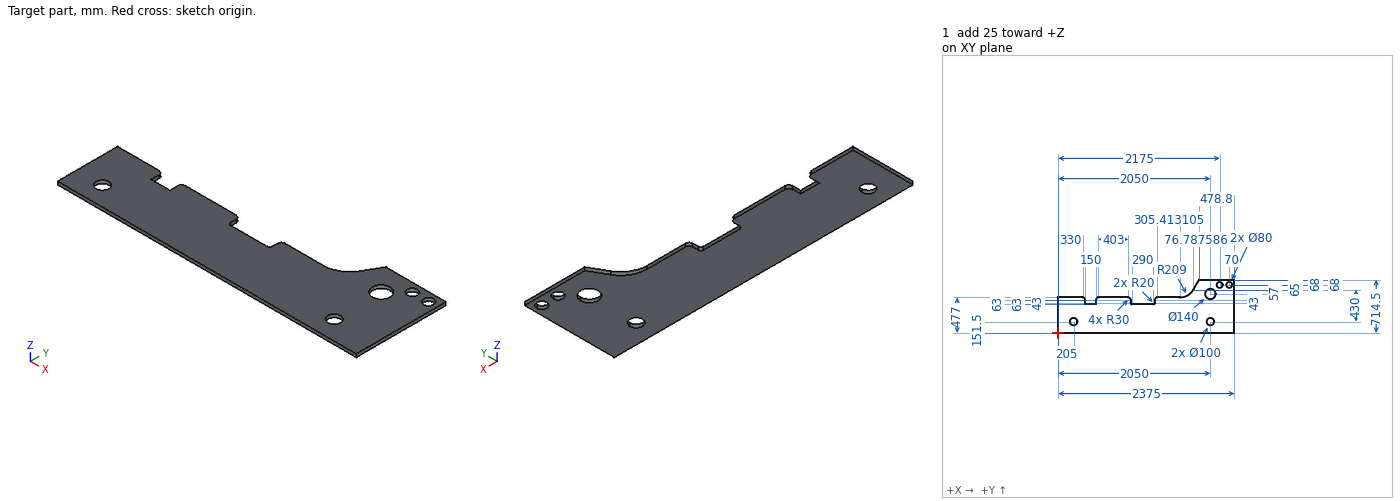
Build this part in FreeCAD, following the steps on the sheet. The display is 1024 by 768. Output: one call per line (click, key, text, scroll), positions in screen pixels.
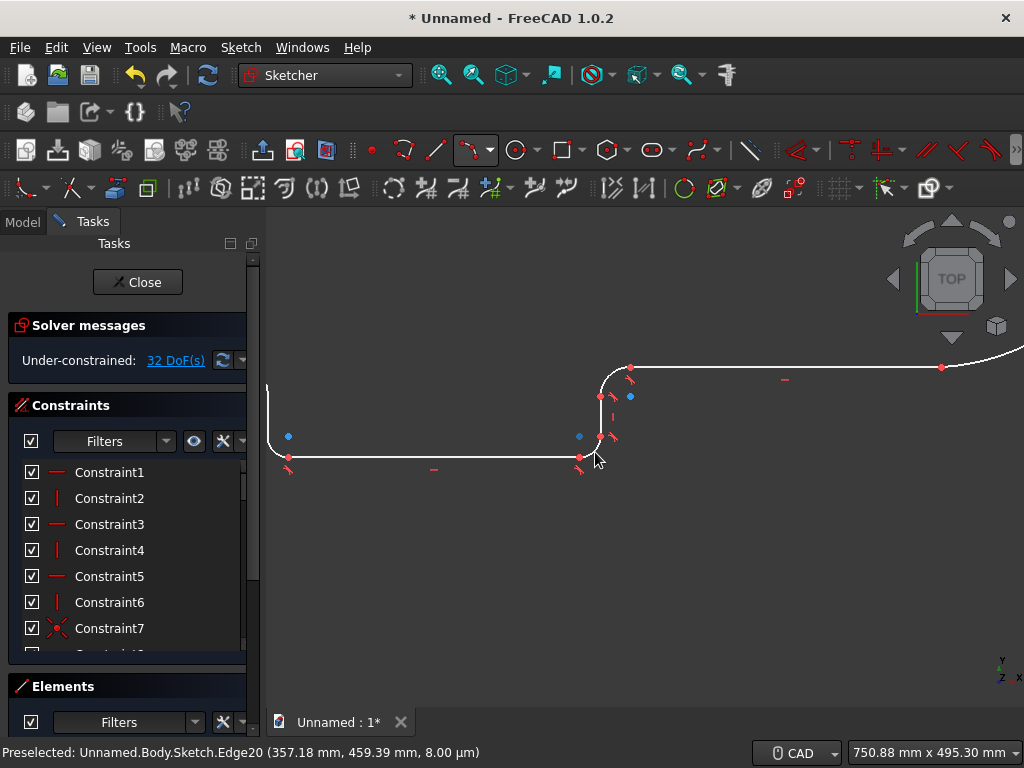
click(594, 451)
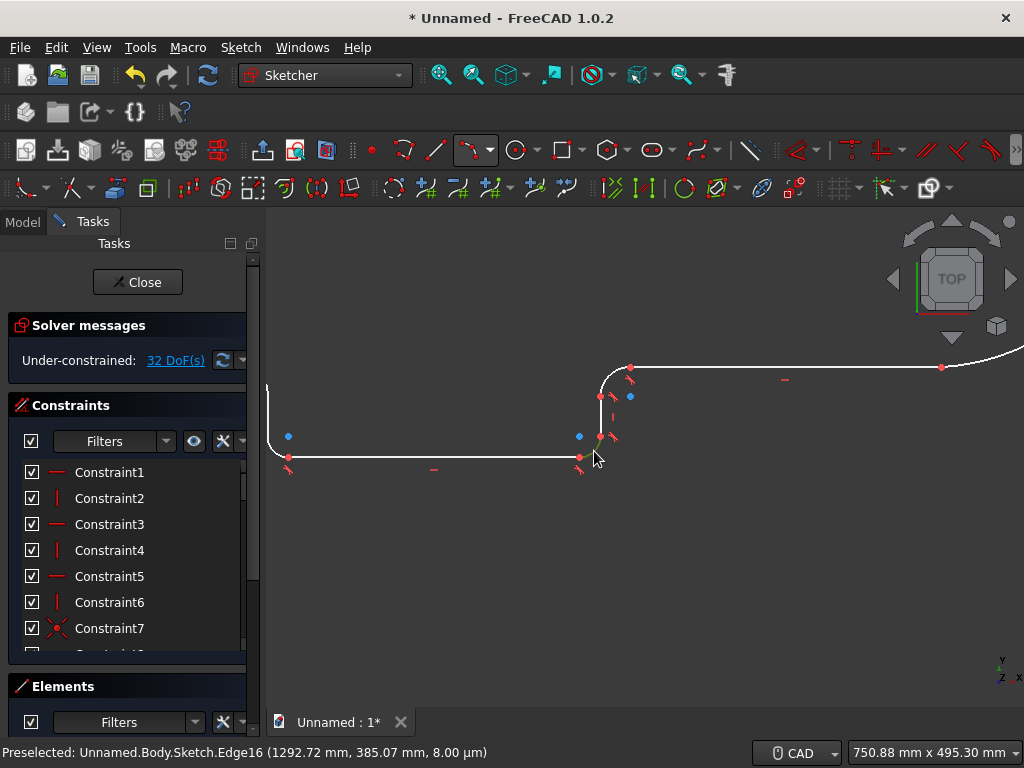
scroll(595, 452, down, 9)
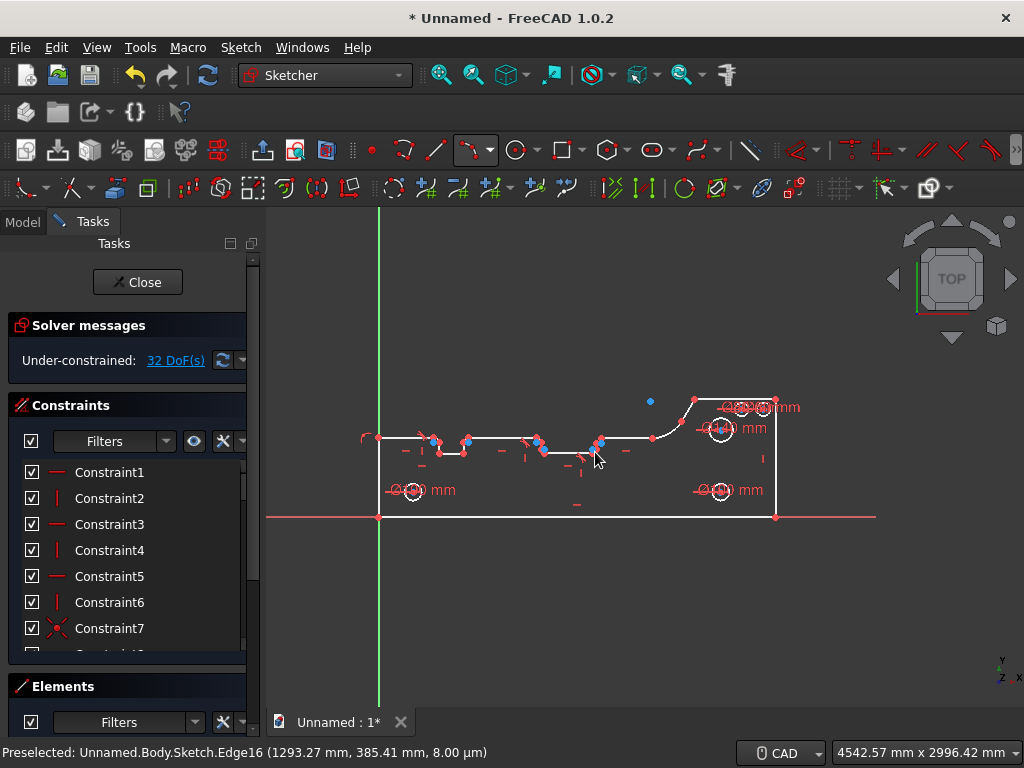
scroll(542, 451, up, 11)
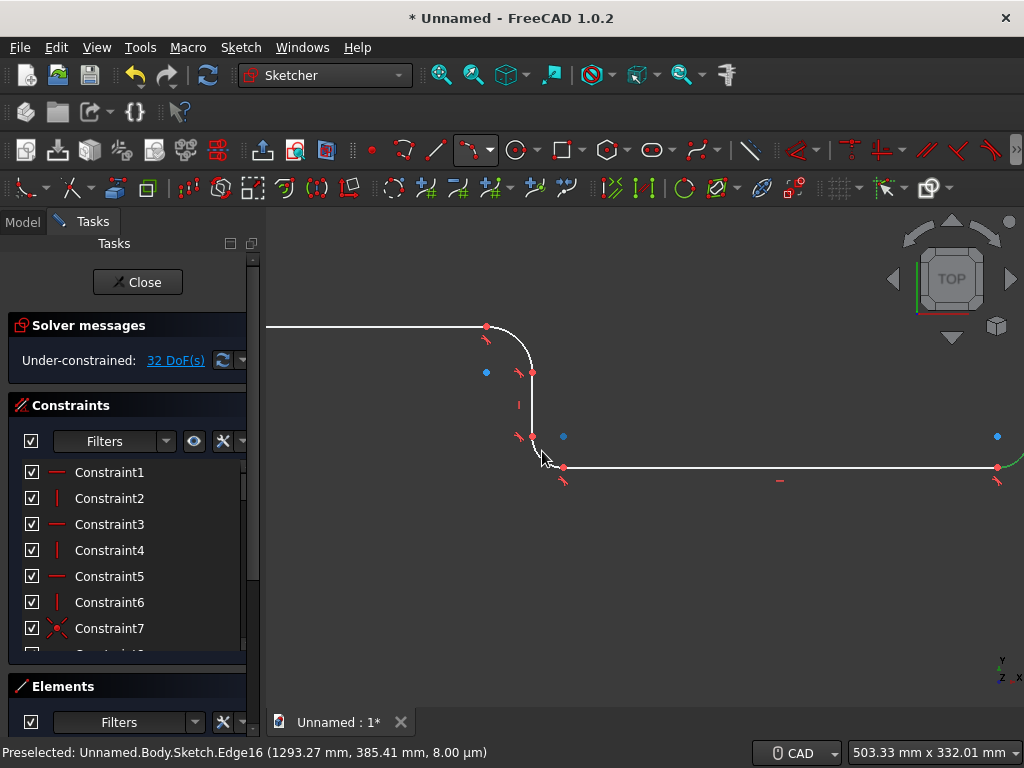
click(536, 451)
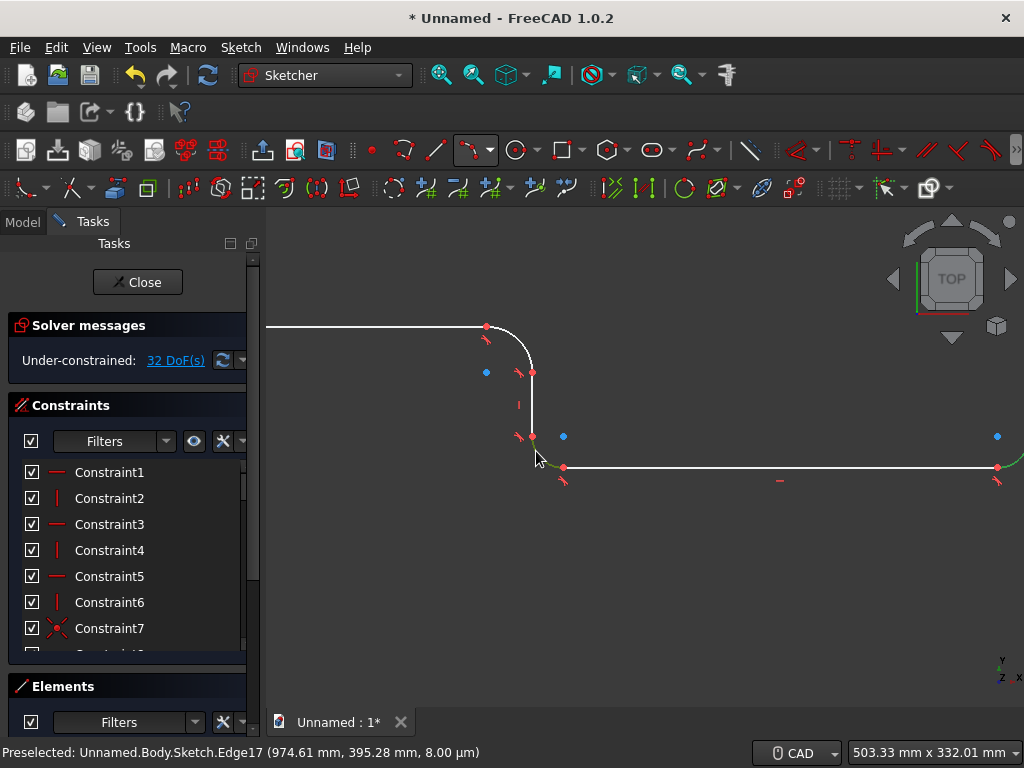
key(e)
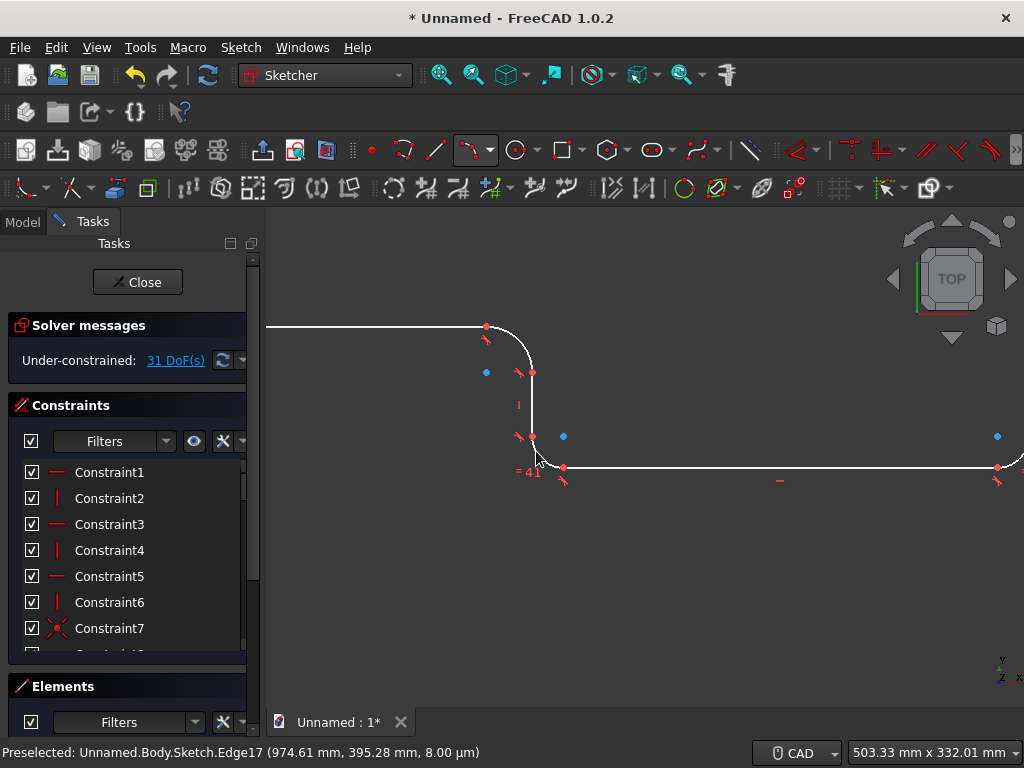
scroll(542, 451, down, 11)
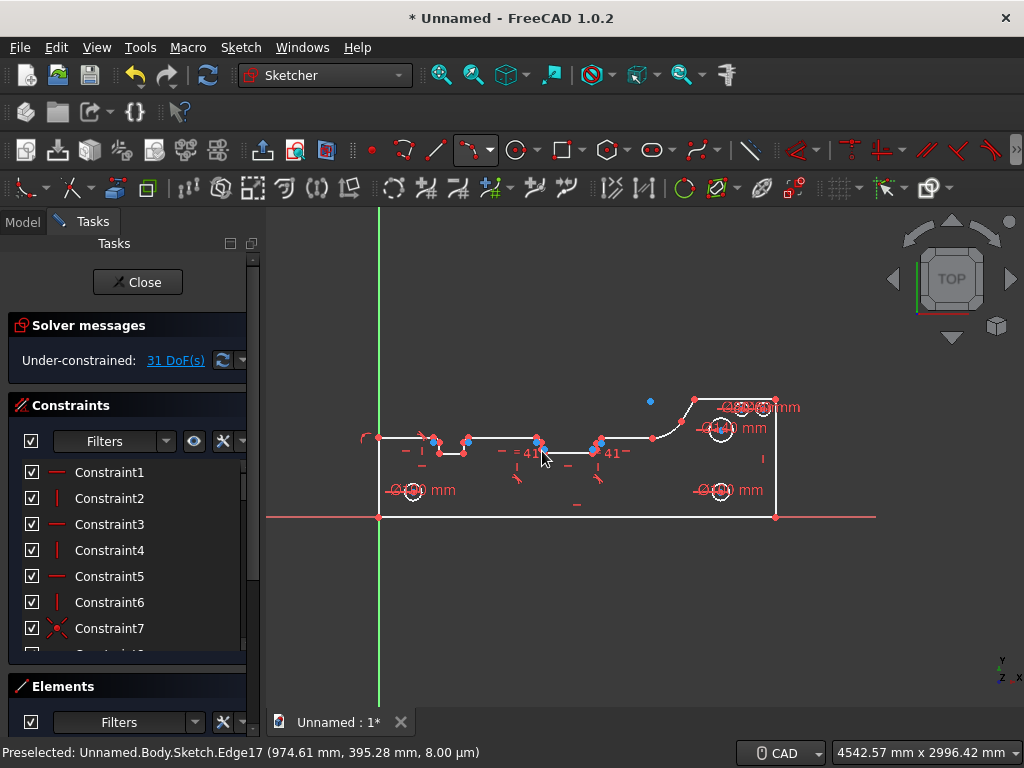
scroll(599, 439, up, 9)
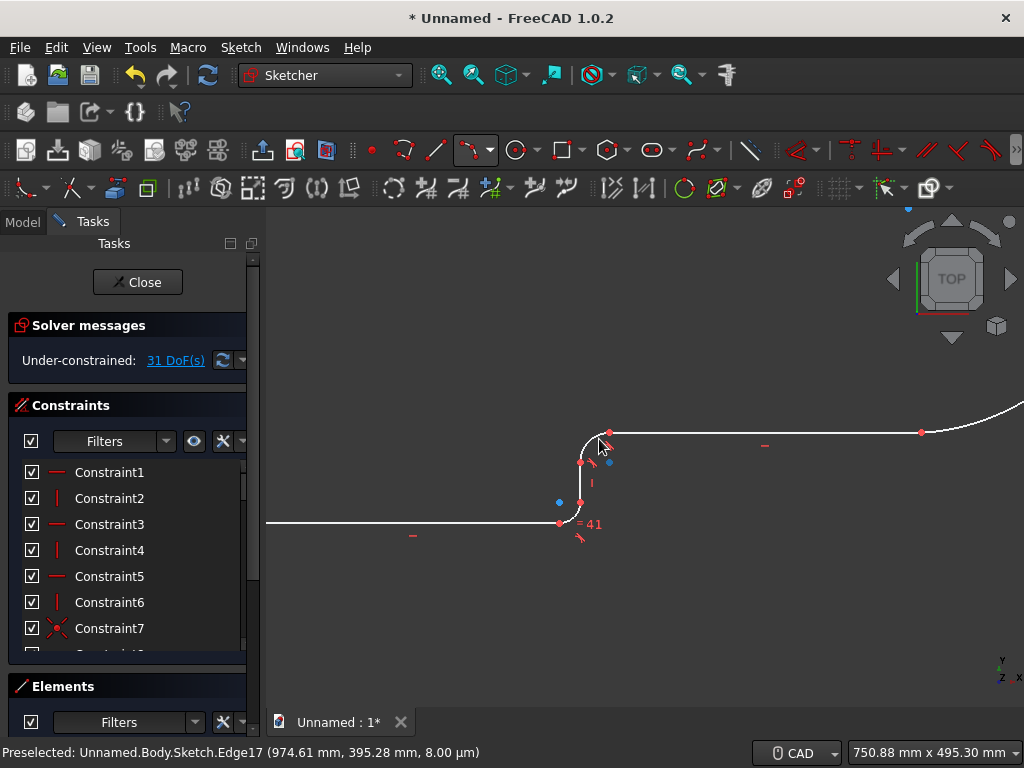
click(597, 436)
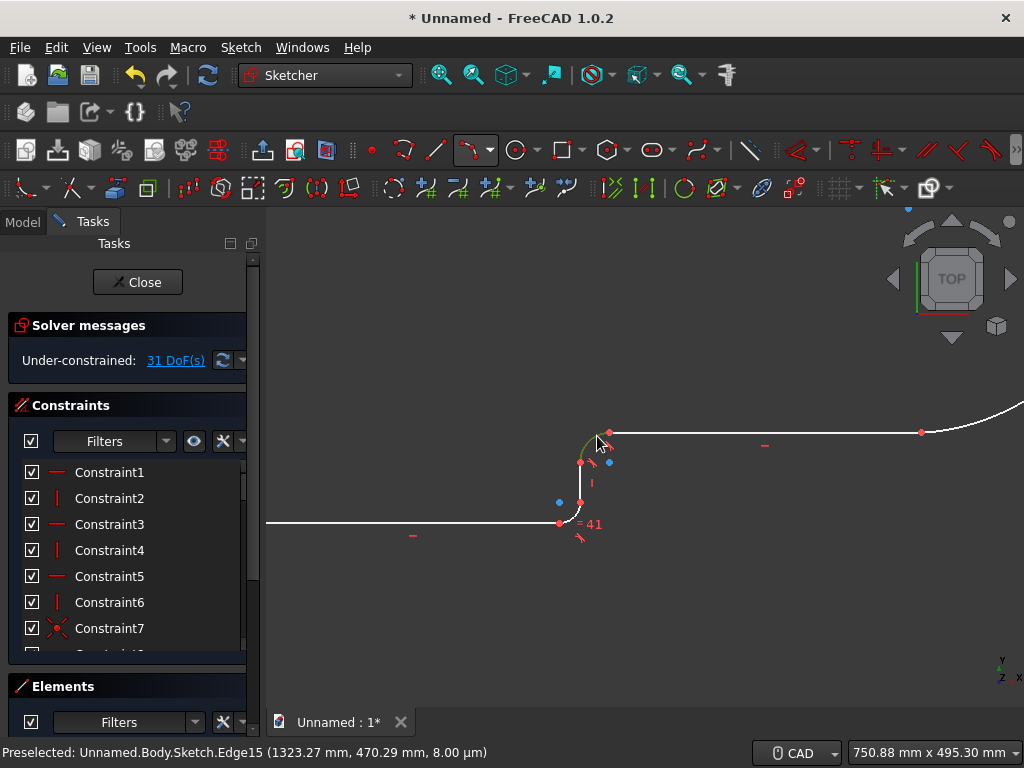
scroll(599, 439, down, 9)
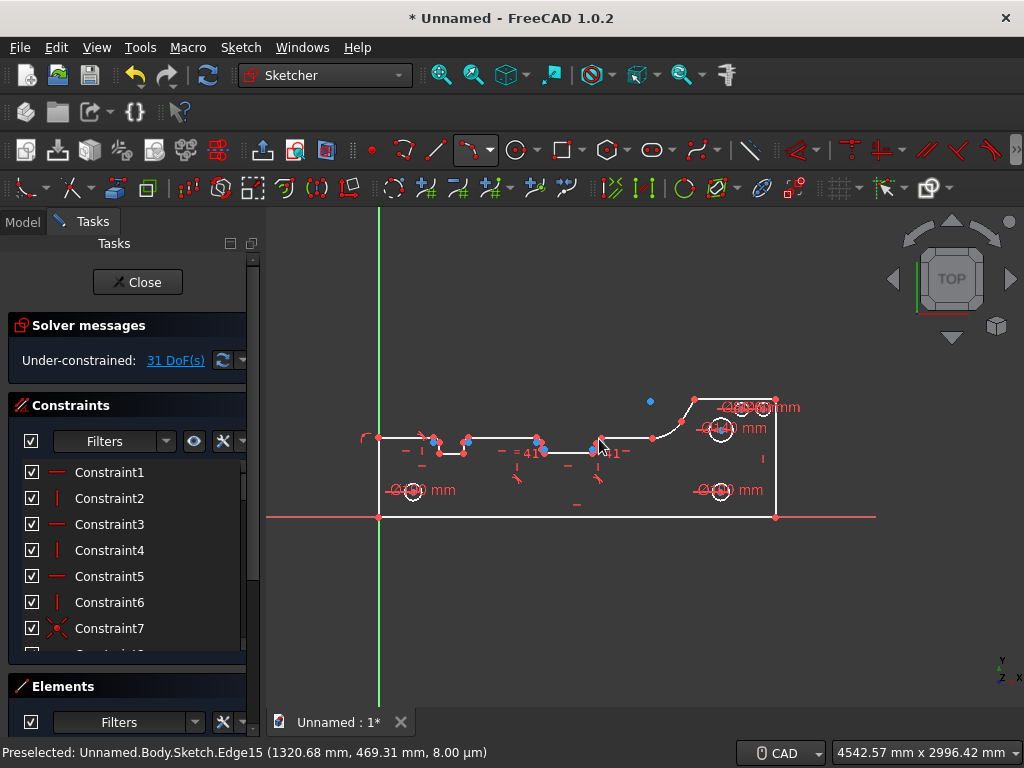
scroll(541, 440, up, 9)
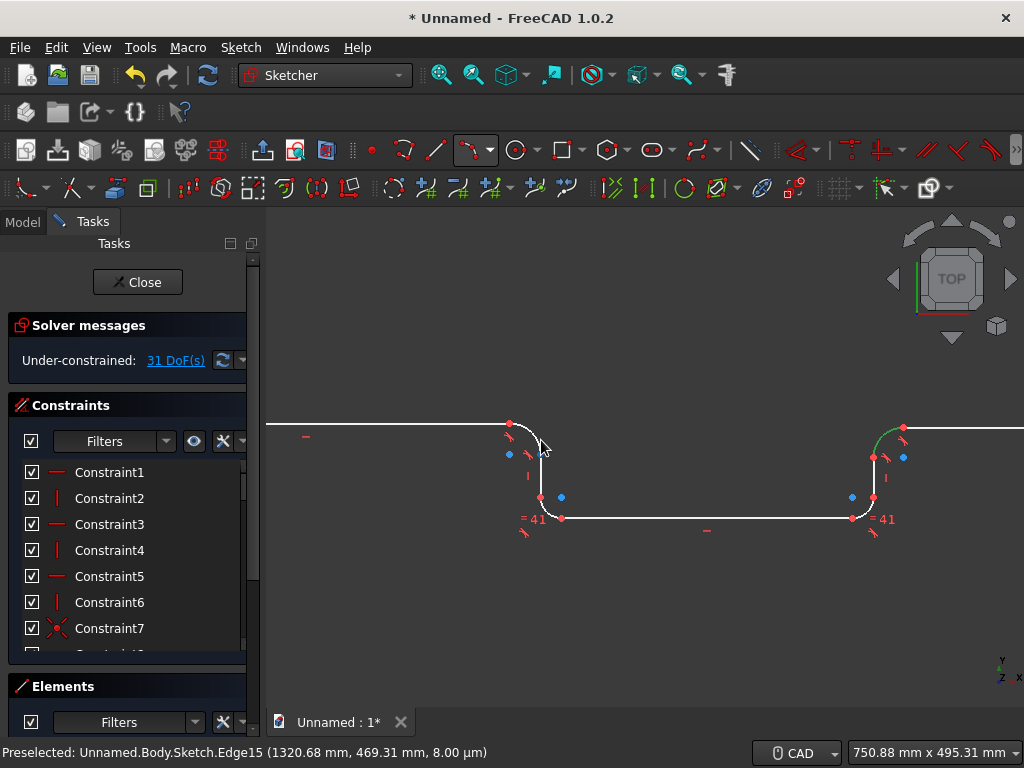
click(537, 440)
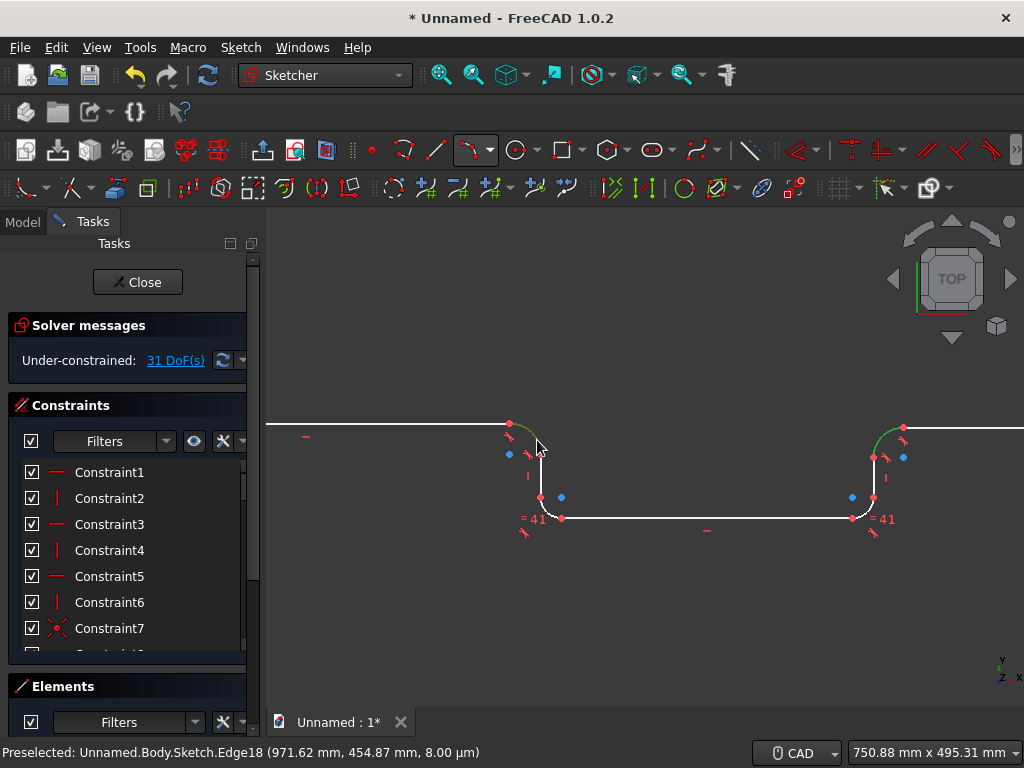
scroll(541, 440, down, 9)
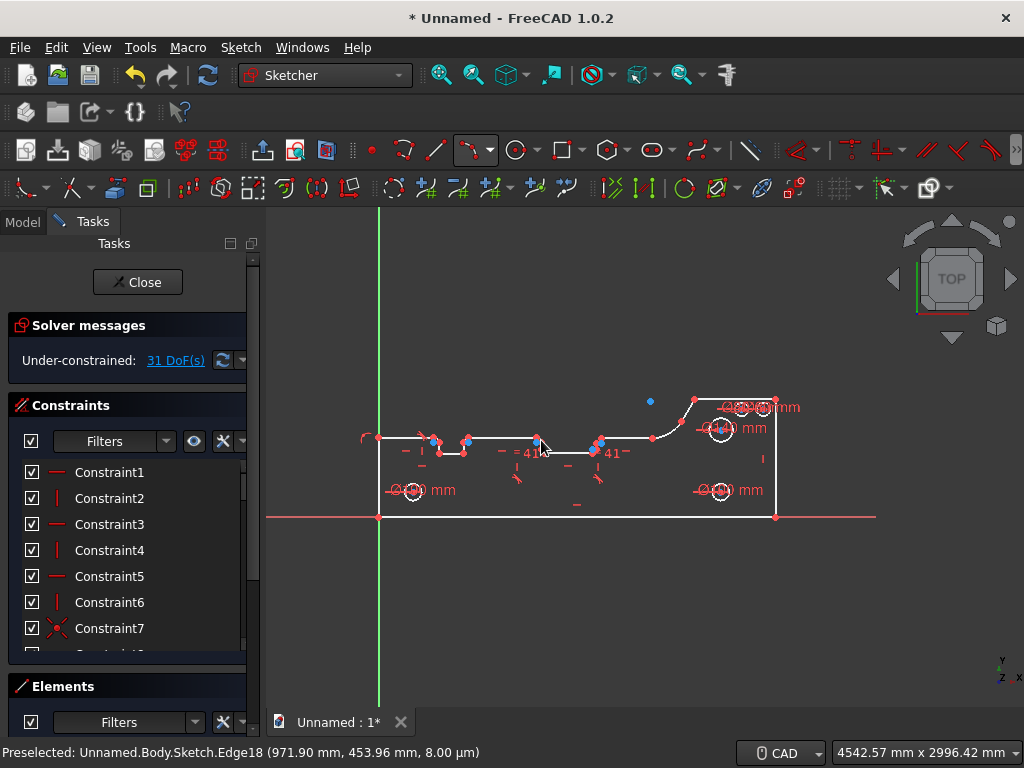
scroll(466, 438, up, 9)